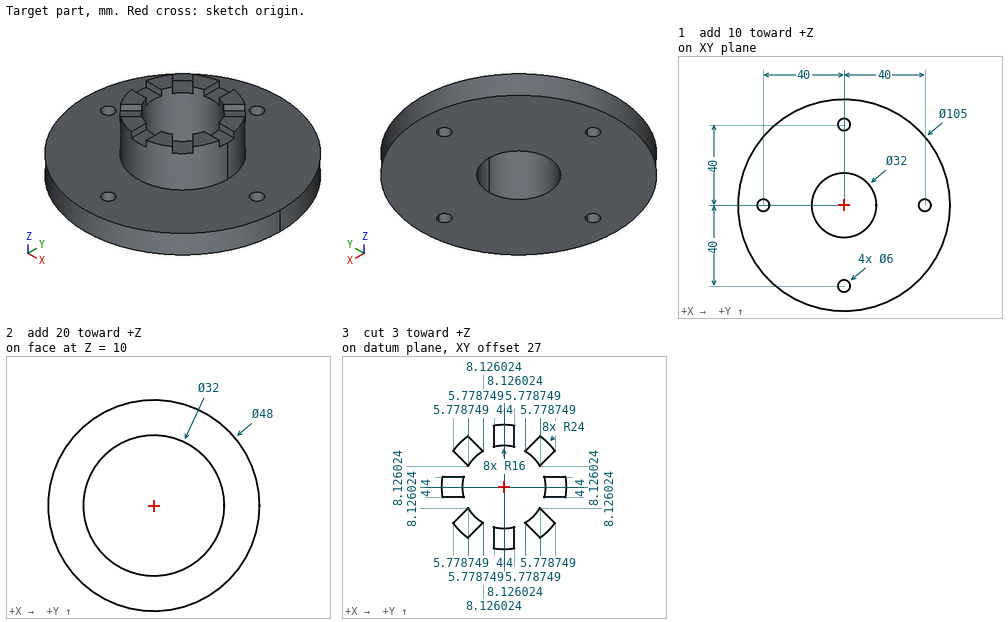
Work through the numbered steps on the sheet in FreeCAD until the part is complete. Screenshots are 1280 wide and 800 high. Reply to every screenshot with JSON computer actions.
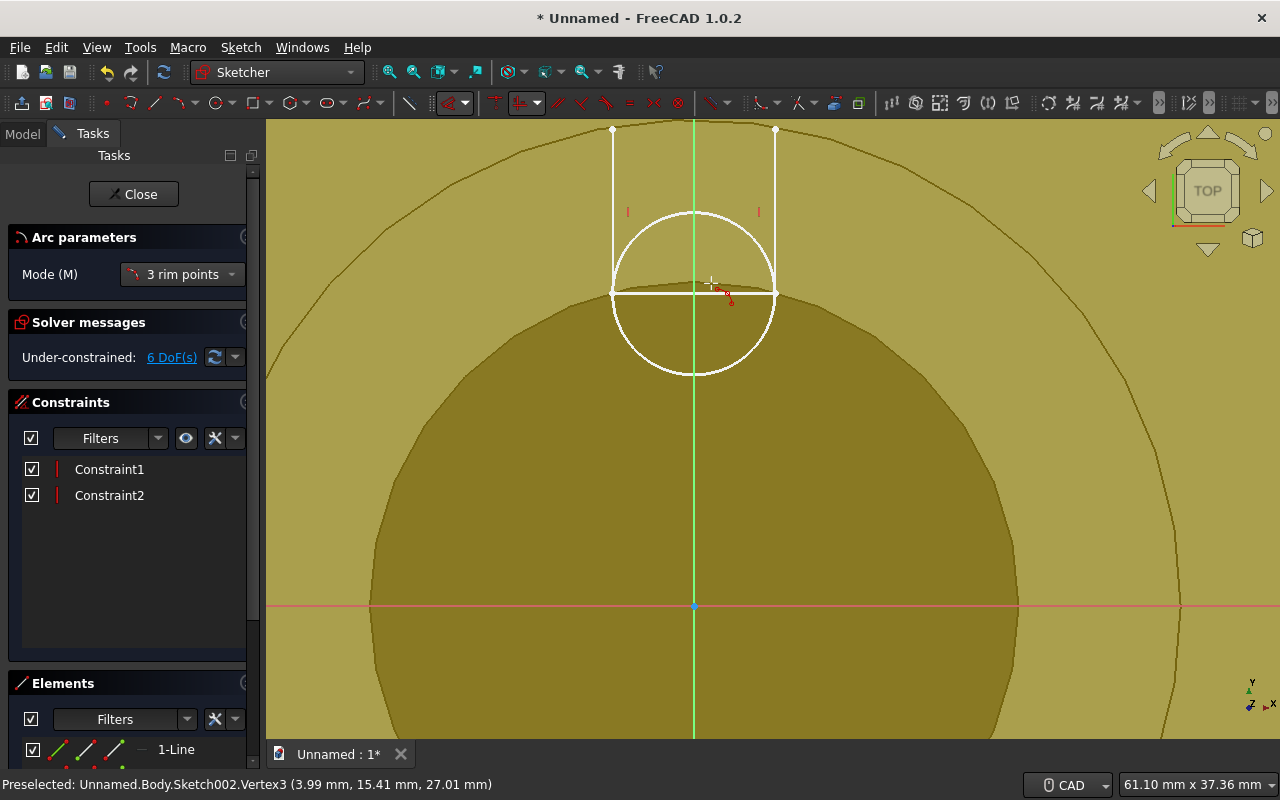
{"action": "left_click", "coordinate": [710, 282]}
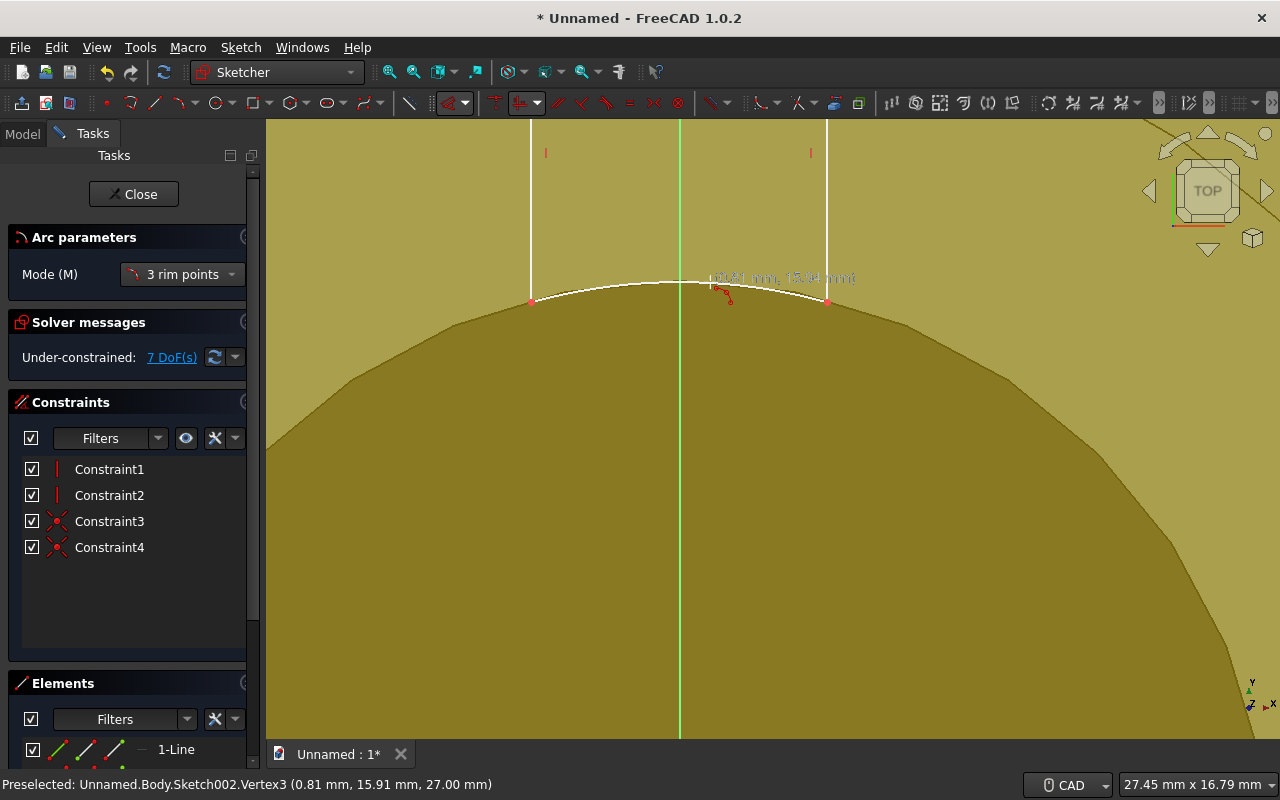
{"action": "scroll", "coordinate": [713, 284], "scroll_direction": "down", "scroll_amount": 7}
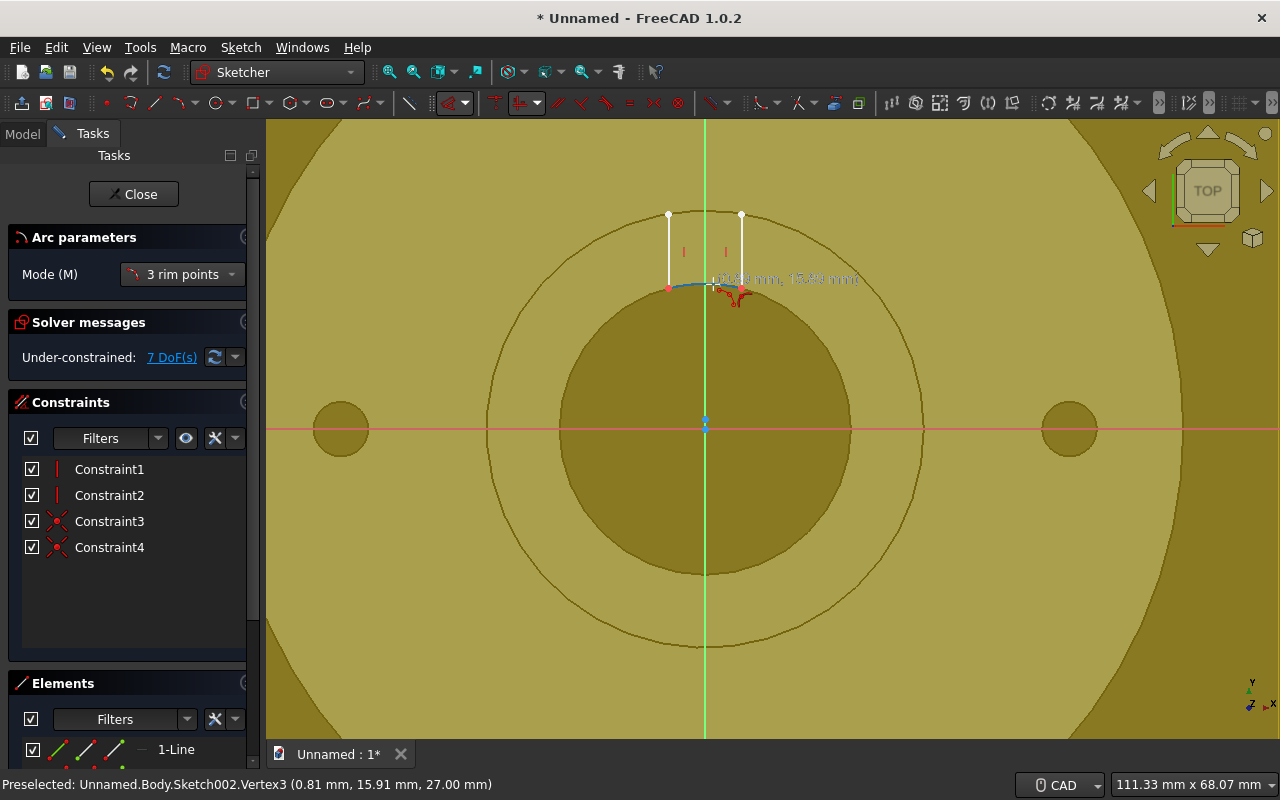
{"action": "left_click", "coordinate": [742, 215]}
{"action": "left_click", "coordinate": [669, 215]}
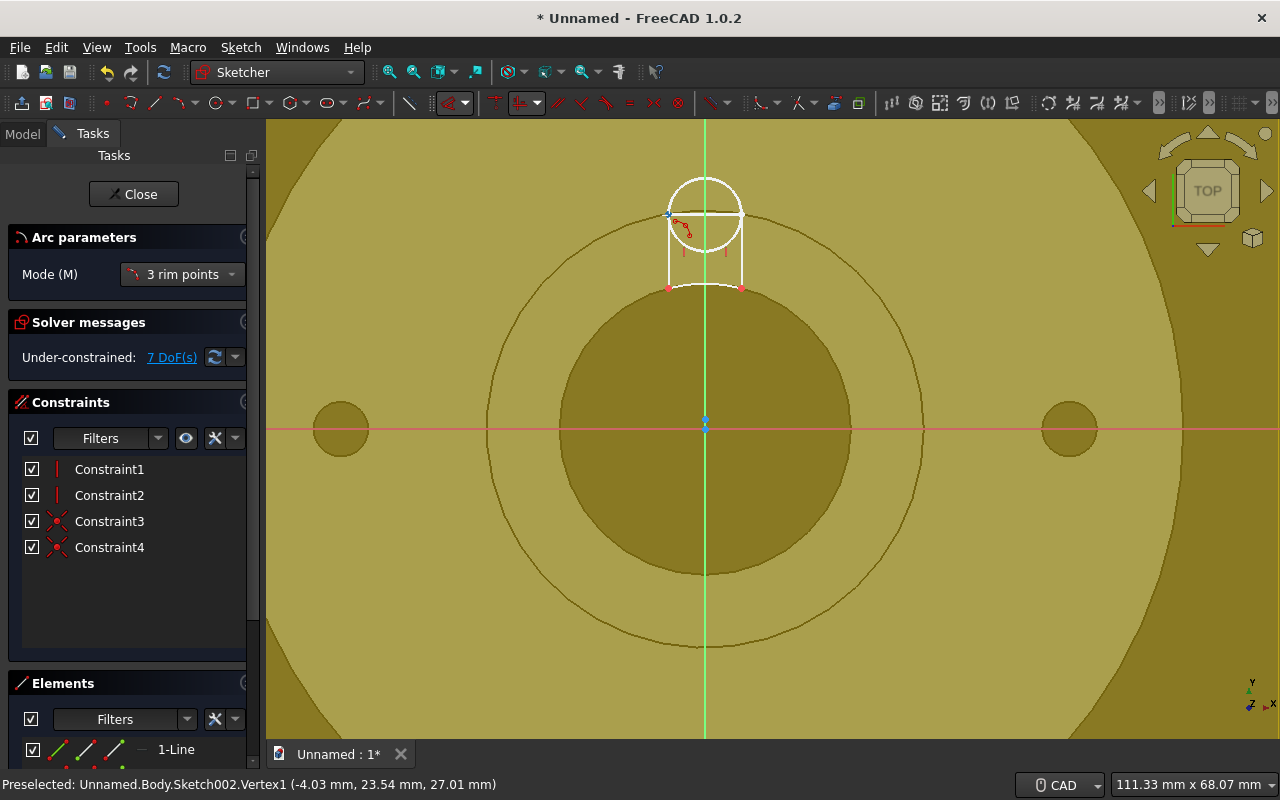
{"action": "scroll", "coordinate": [713, 211], "scroll_direction": "up", "scroll_amount": 9}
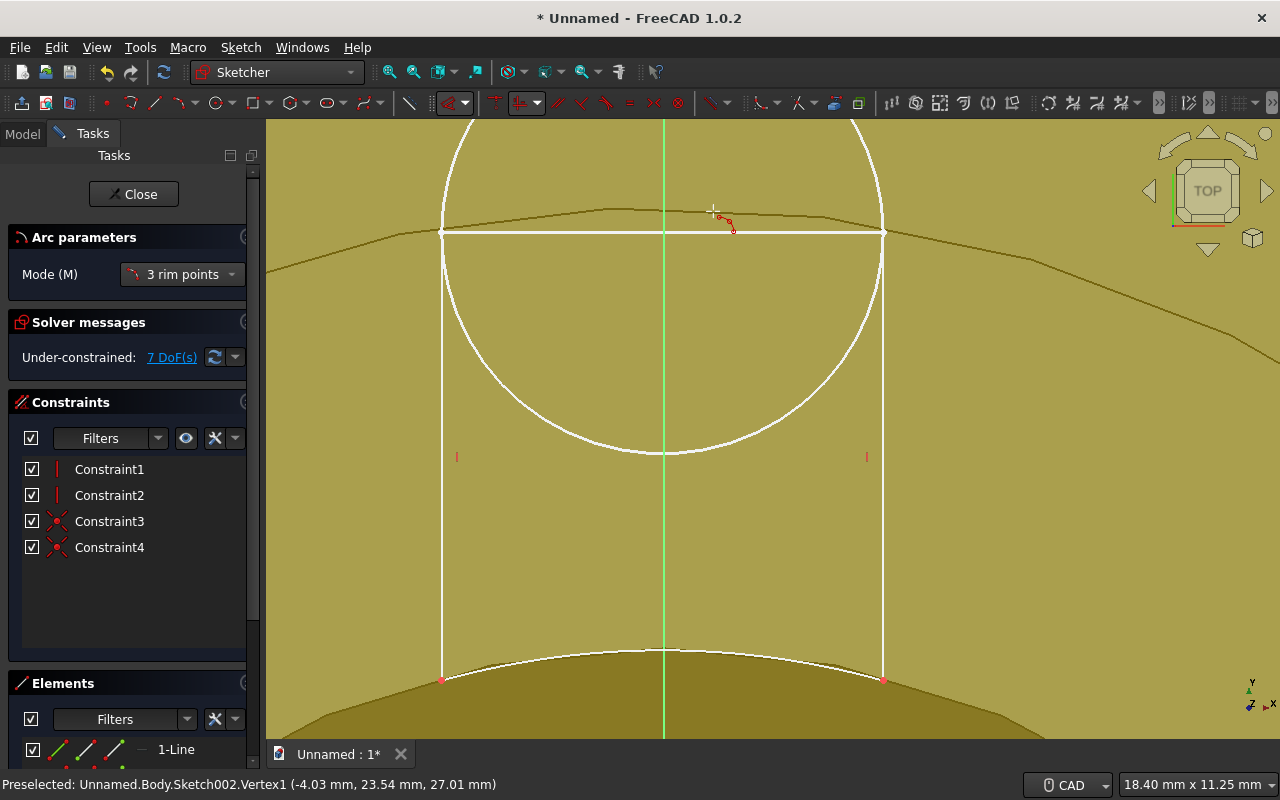
{"action": "left_click", "coordinate": [708, 208]}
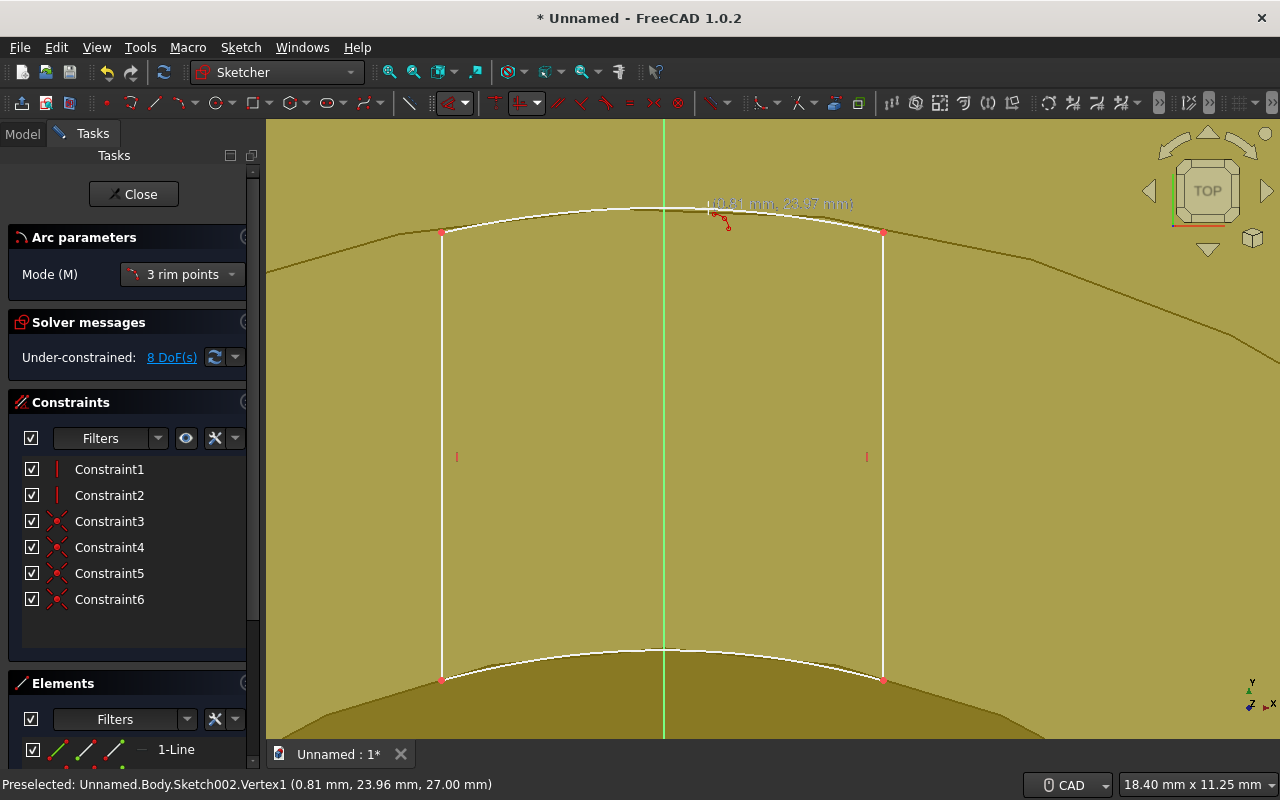
{"action": "left_click", "coordinate": [156, 104]}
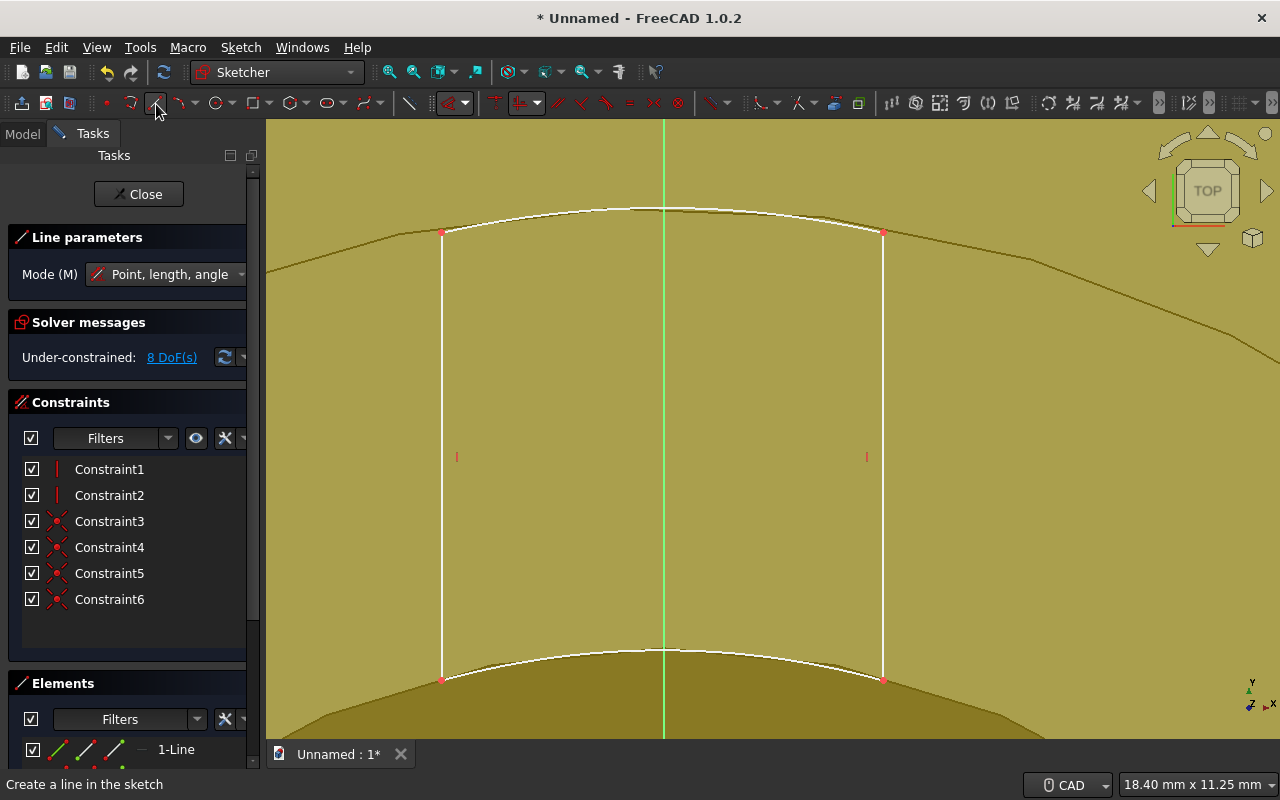
{"action": "scroll", "coordinate": [713, 211], "scroll_direction": "down", "scroll_amount": 9}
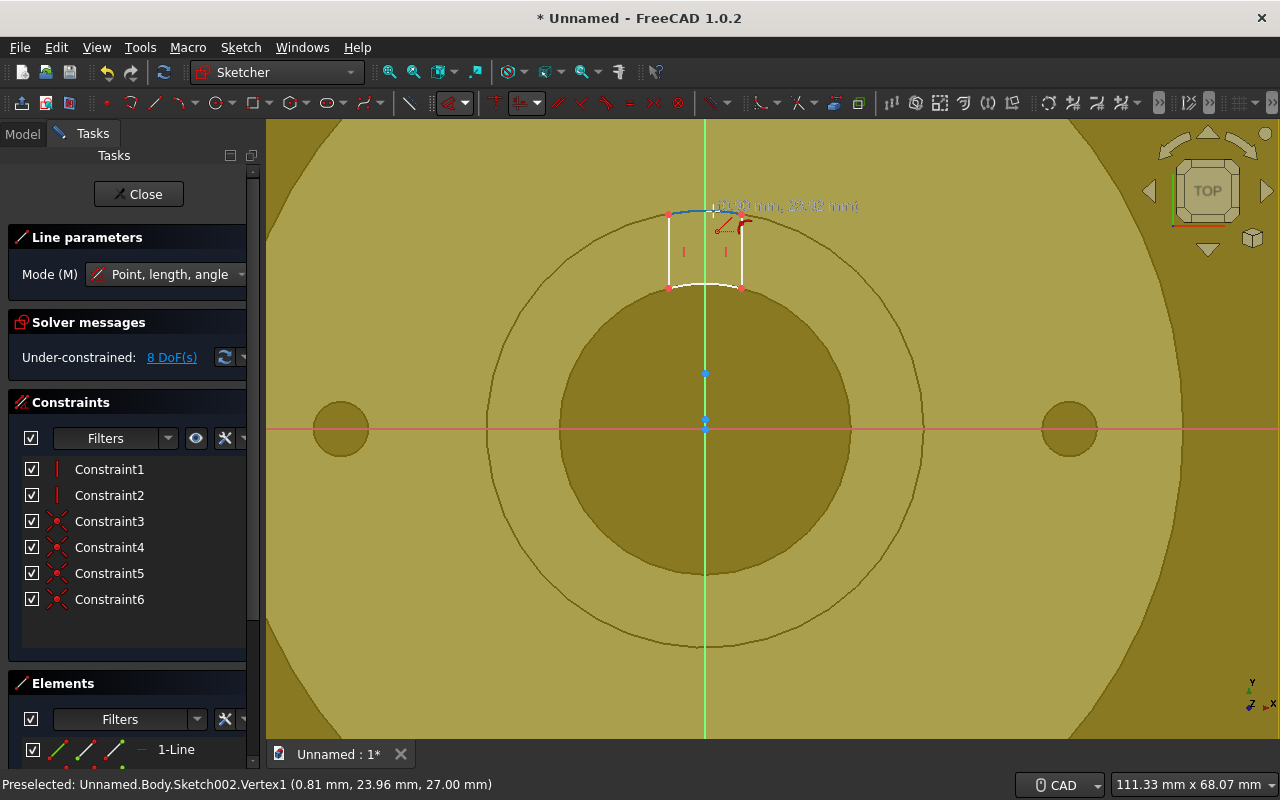
{"action": "left_click", "coordinate": [832, 251]}
{"action": "left_click", "coordinate": [779, 304]}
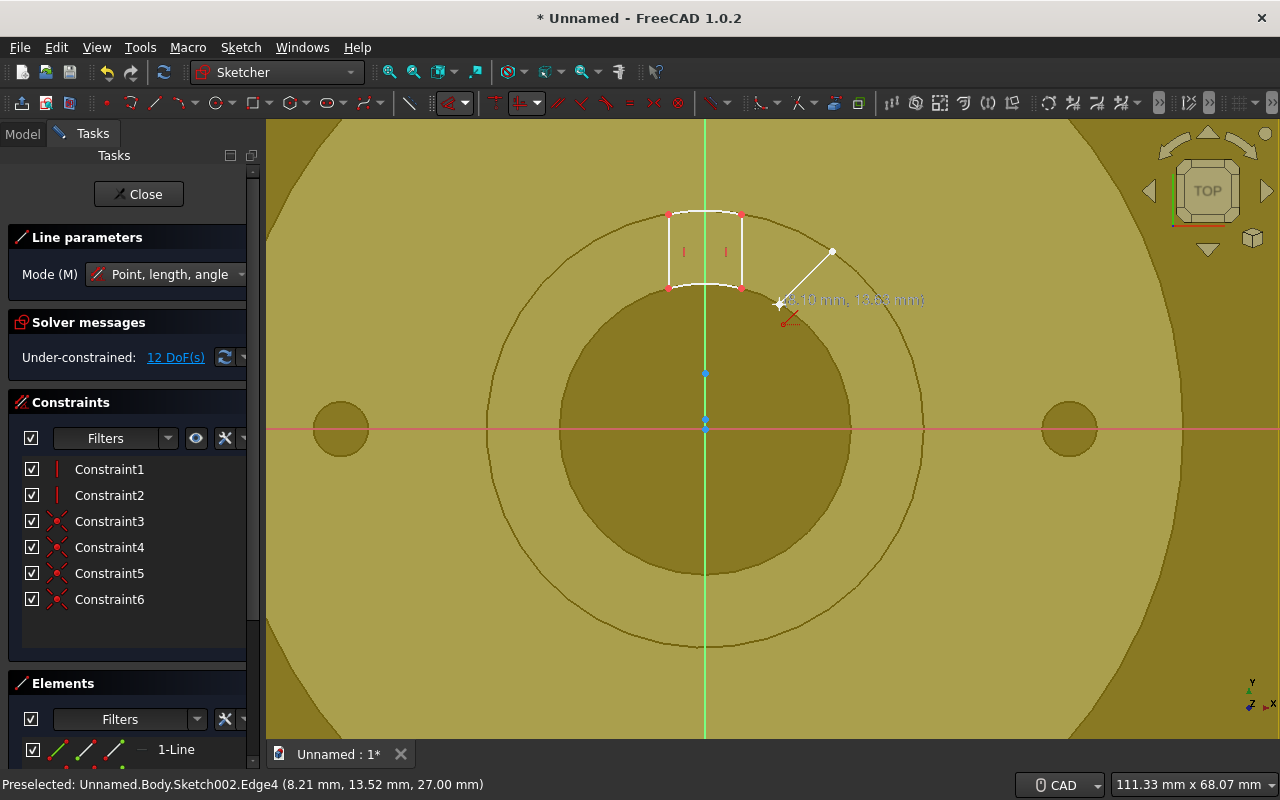
{"action": "left_click", "coordinate": [831, 355]}
{"action": "left_click", "coordinate": [883, 302]}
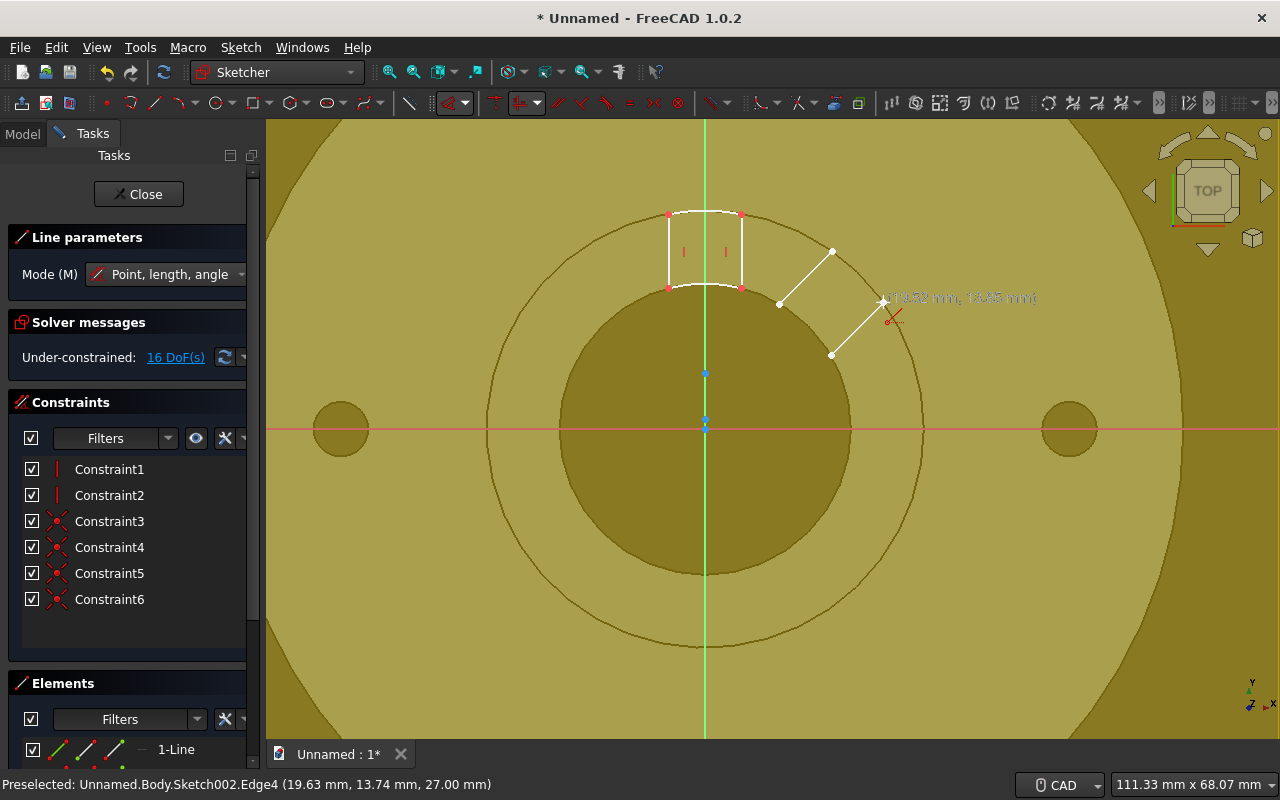
{"action": "left_click", "coordinate": [180, 104]}